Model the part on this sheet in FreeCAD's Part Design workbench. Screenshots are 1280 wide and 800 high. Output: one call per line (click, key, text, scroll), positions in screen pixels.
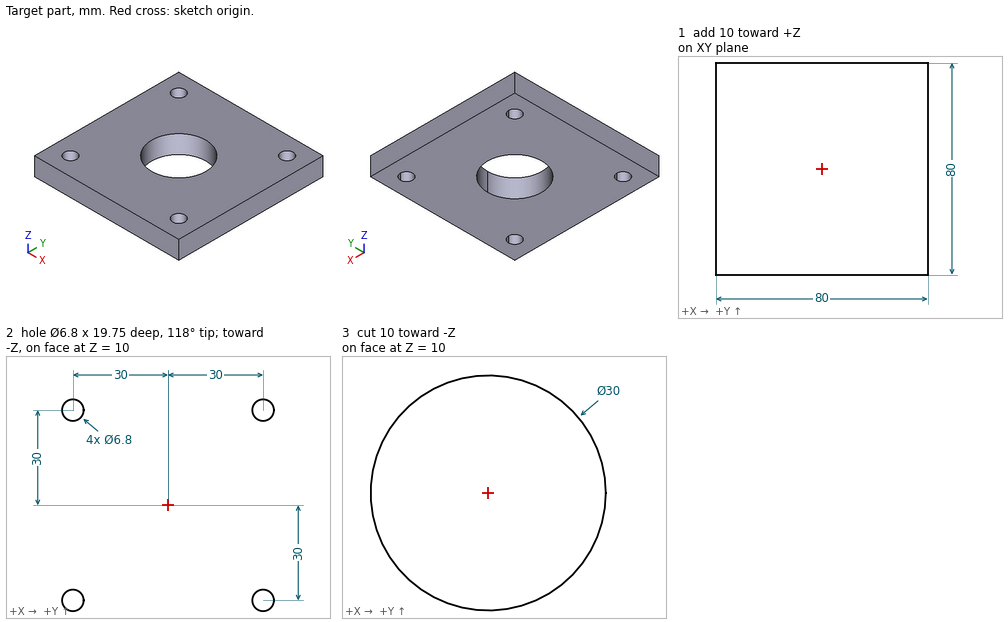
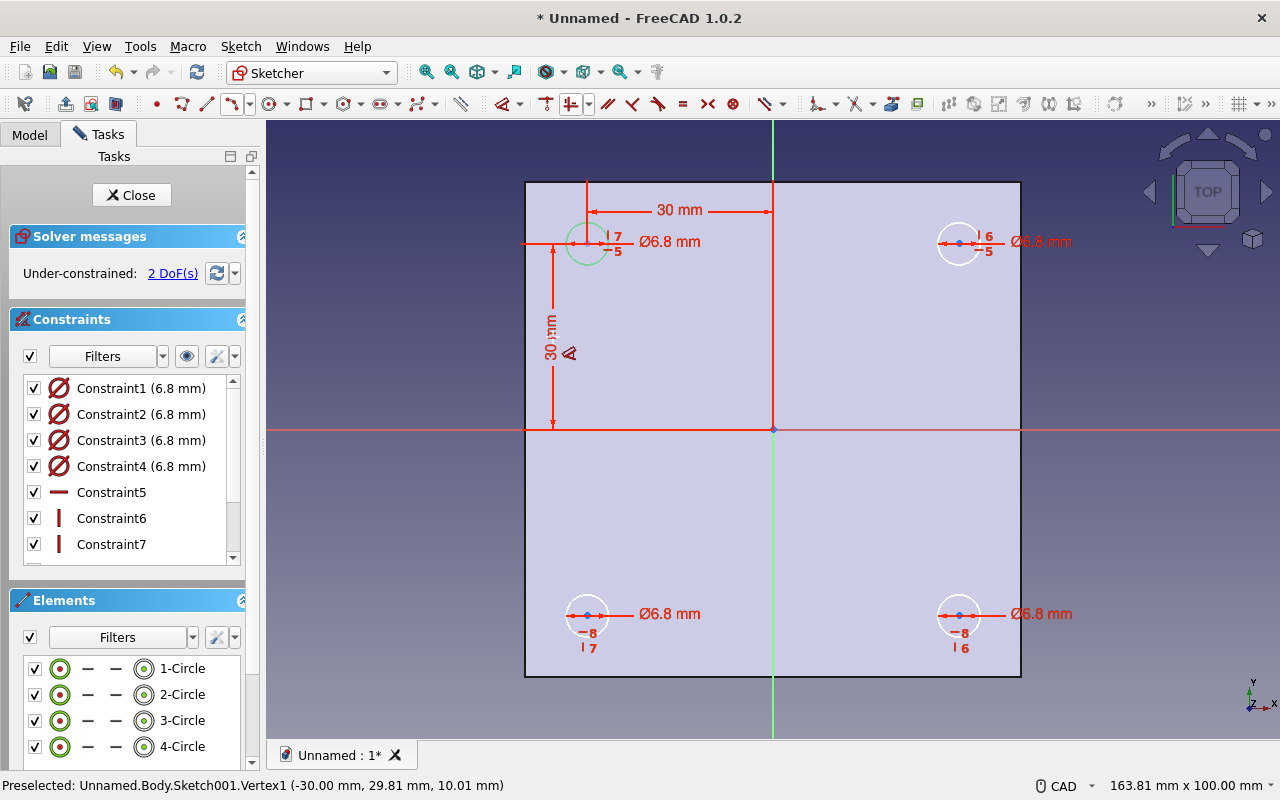
click(959, 244)
click(866, 210)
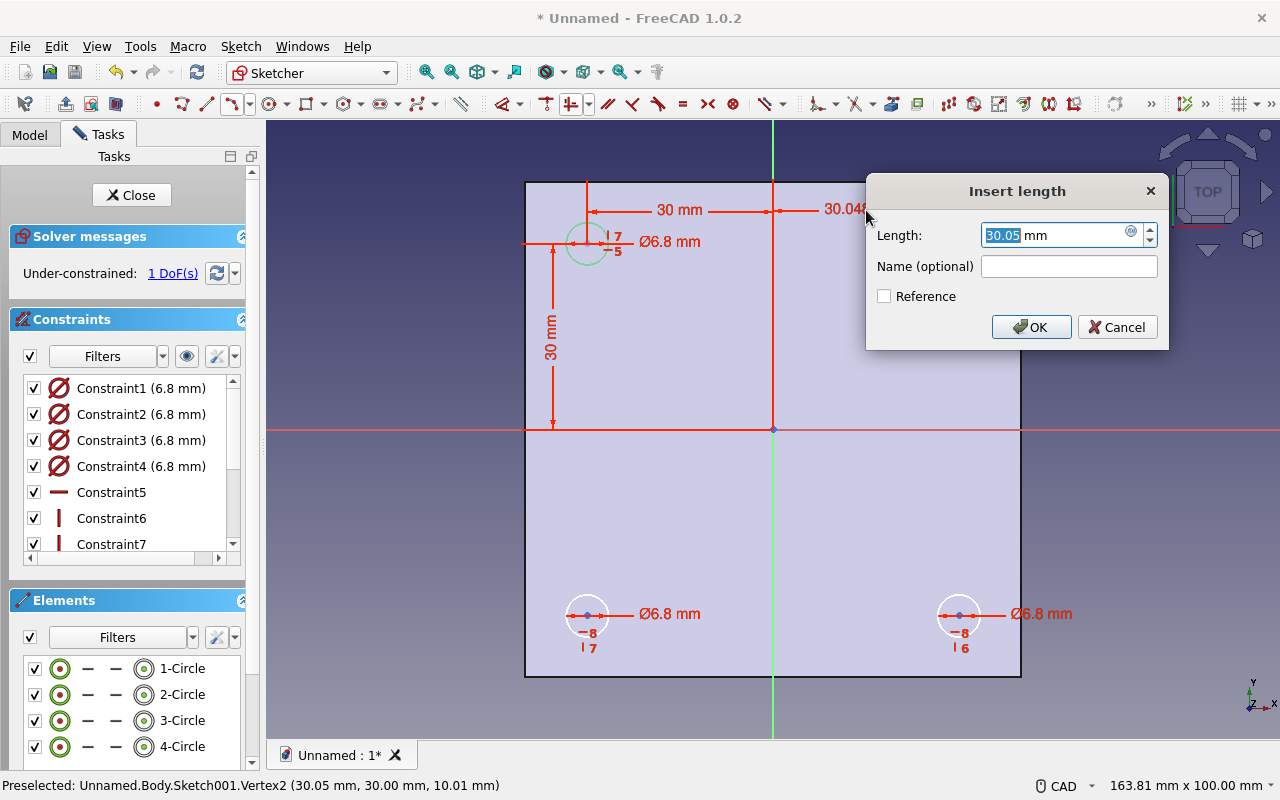
text(30)
key(Return)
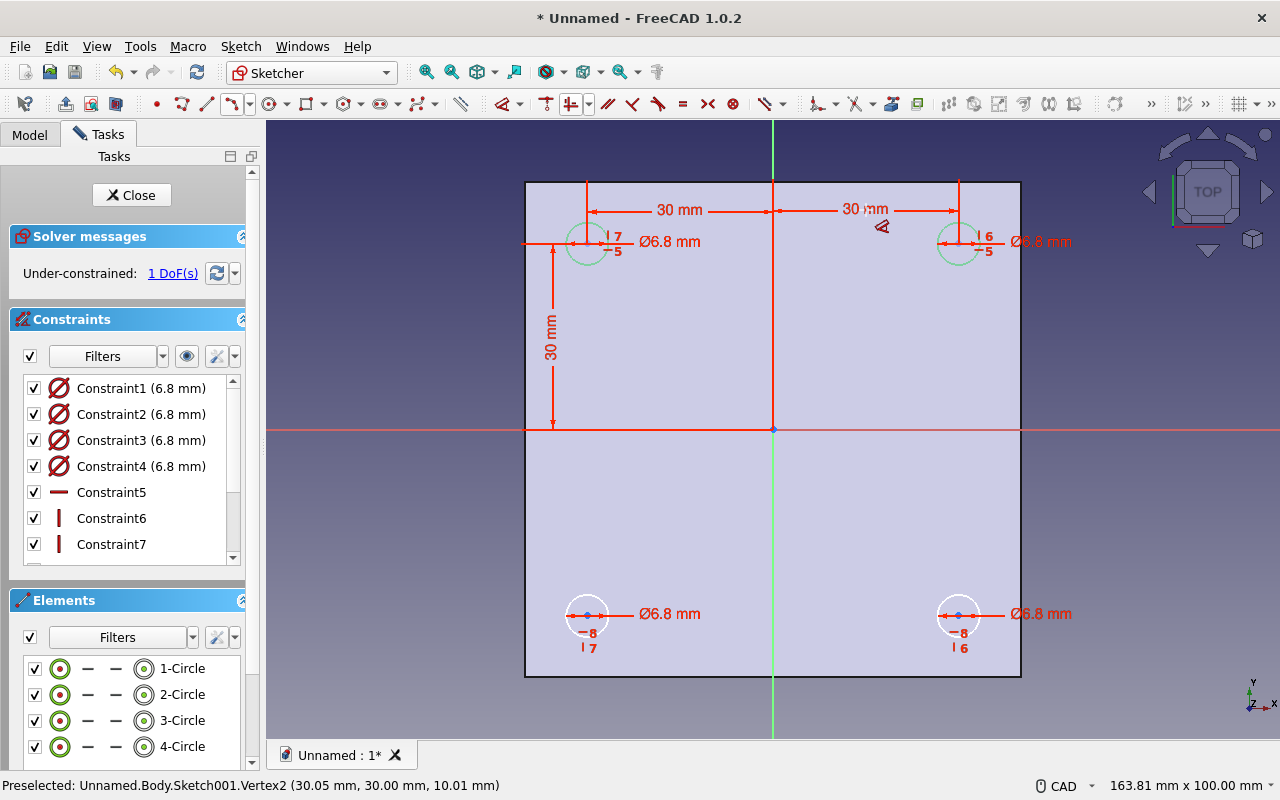
click(959, 616)
click(993, 523)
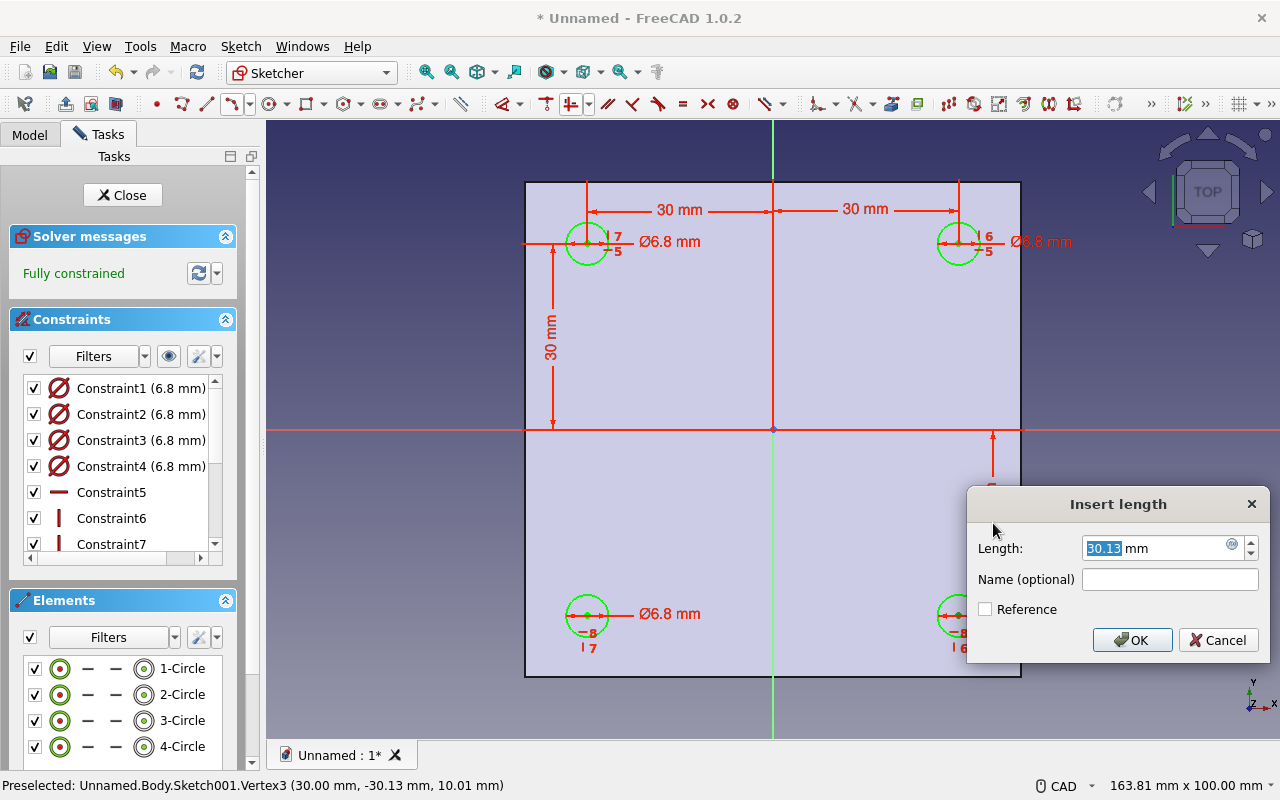
text(30)
key(Return)
key(Escape)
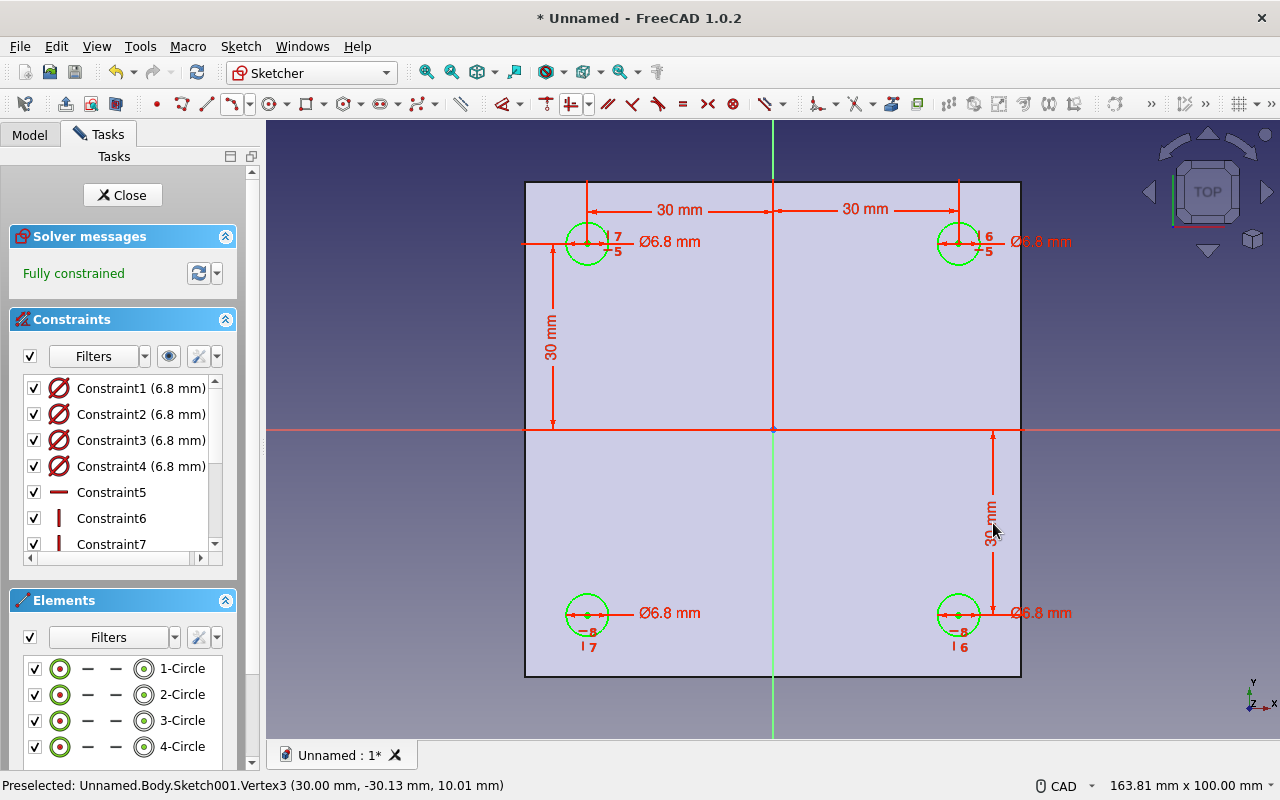
click(123, 195)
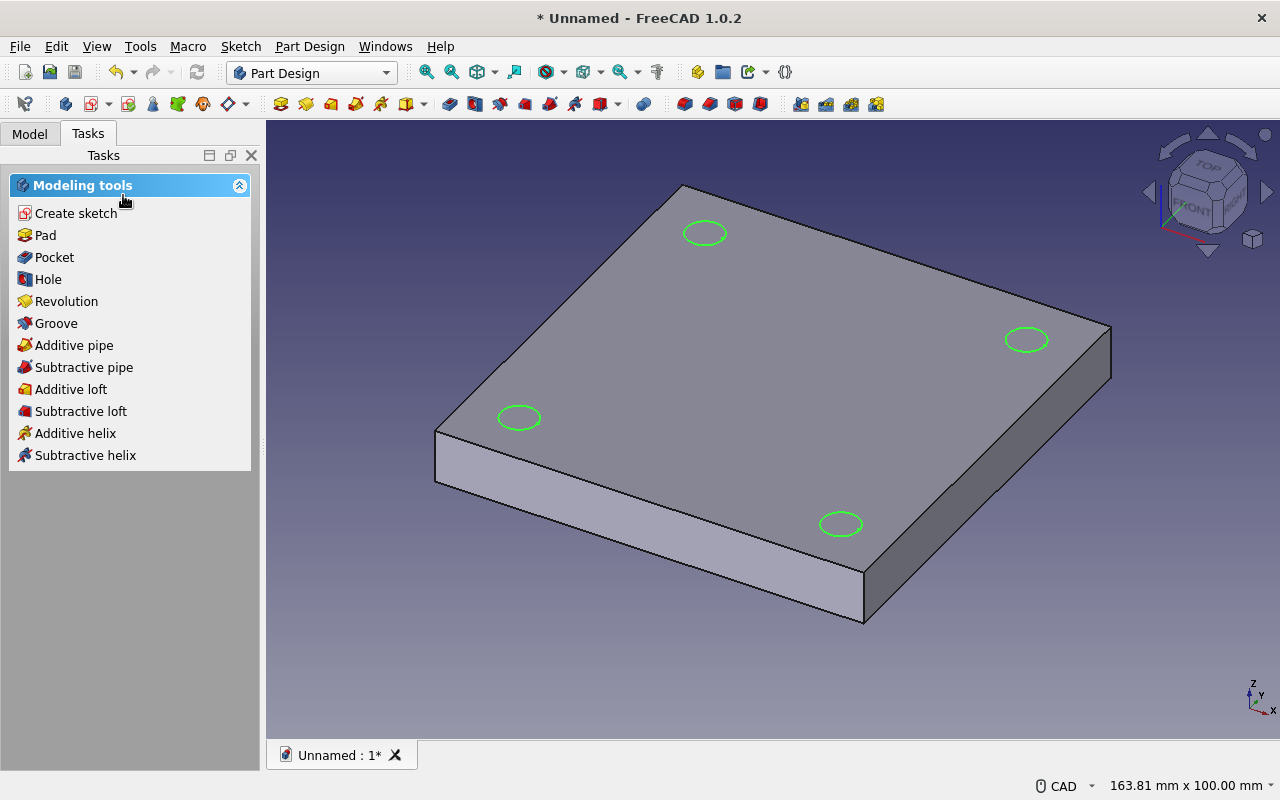
click(475, 104)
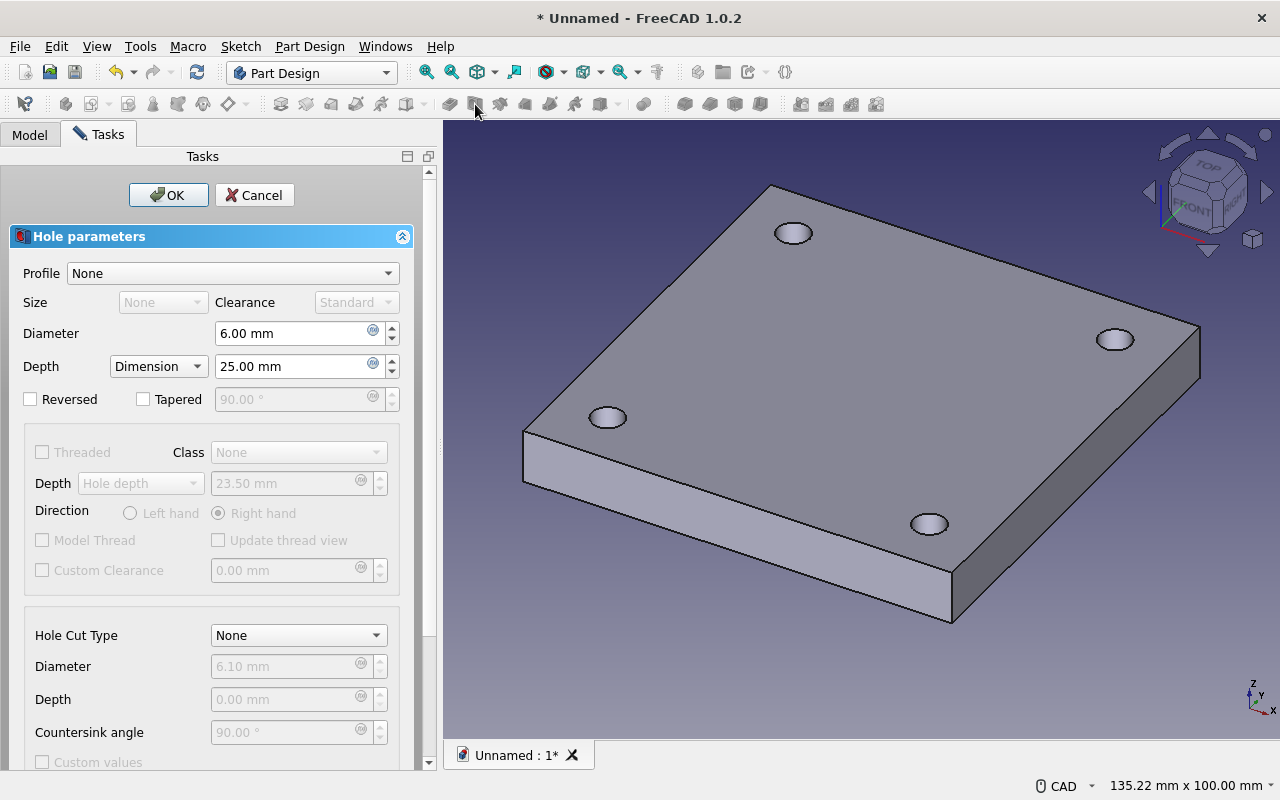
triple_click(300, 334)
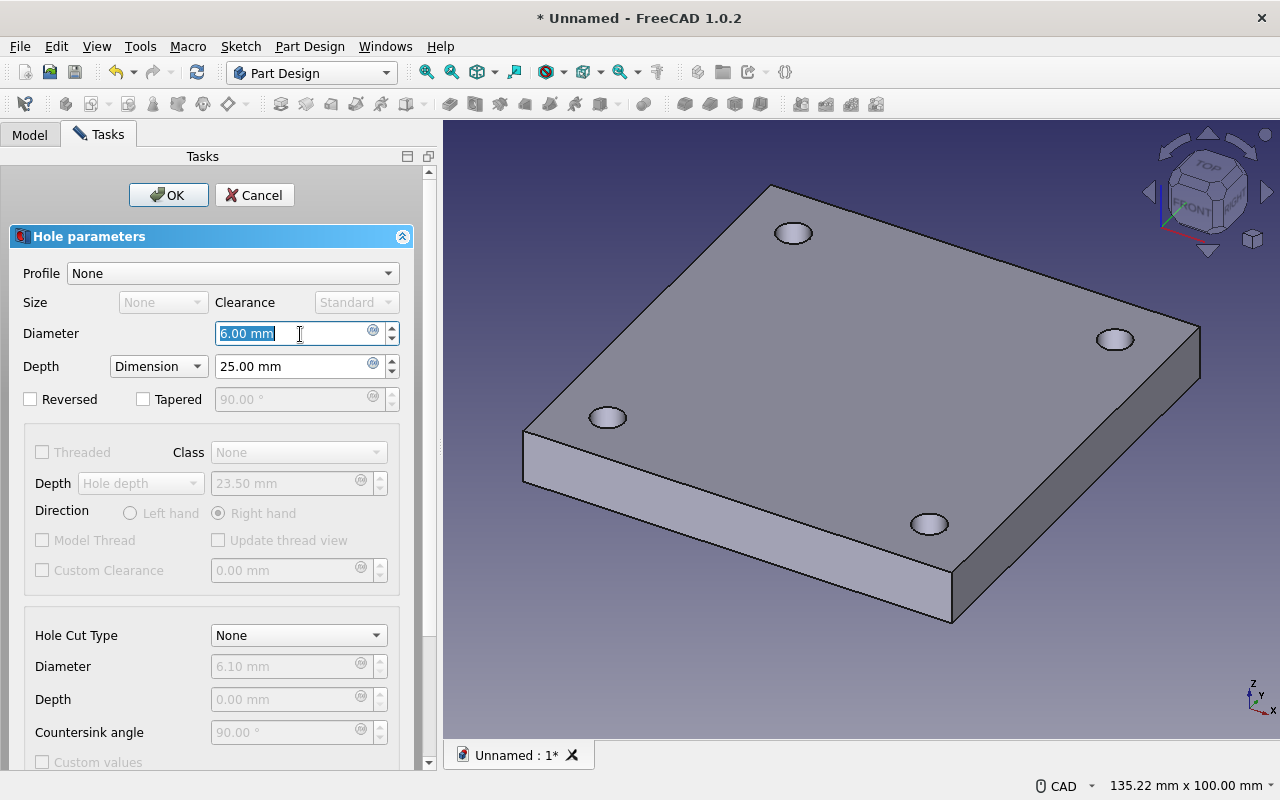
text(6.8)
key(Tab)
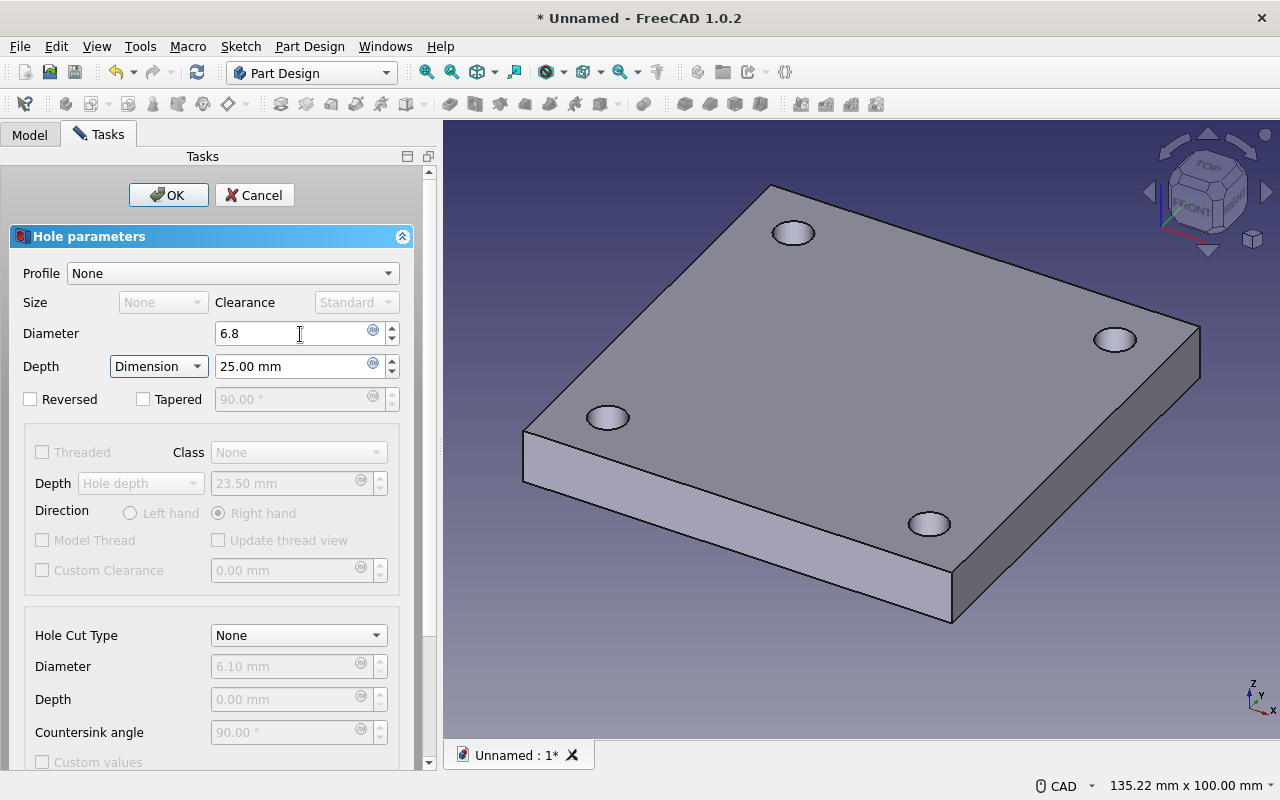
triple_click(300, 366)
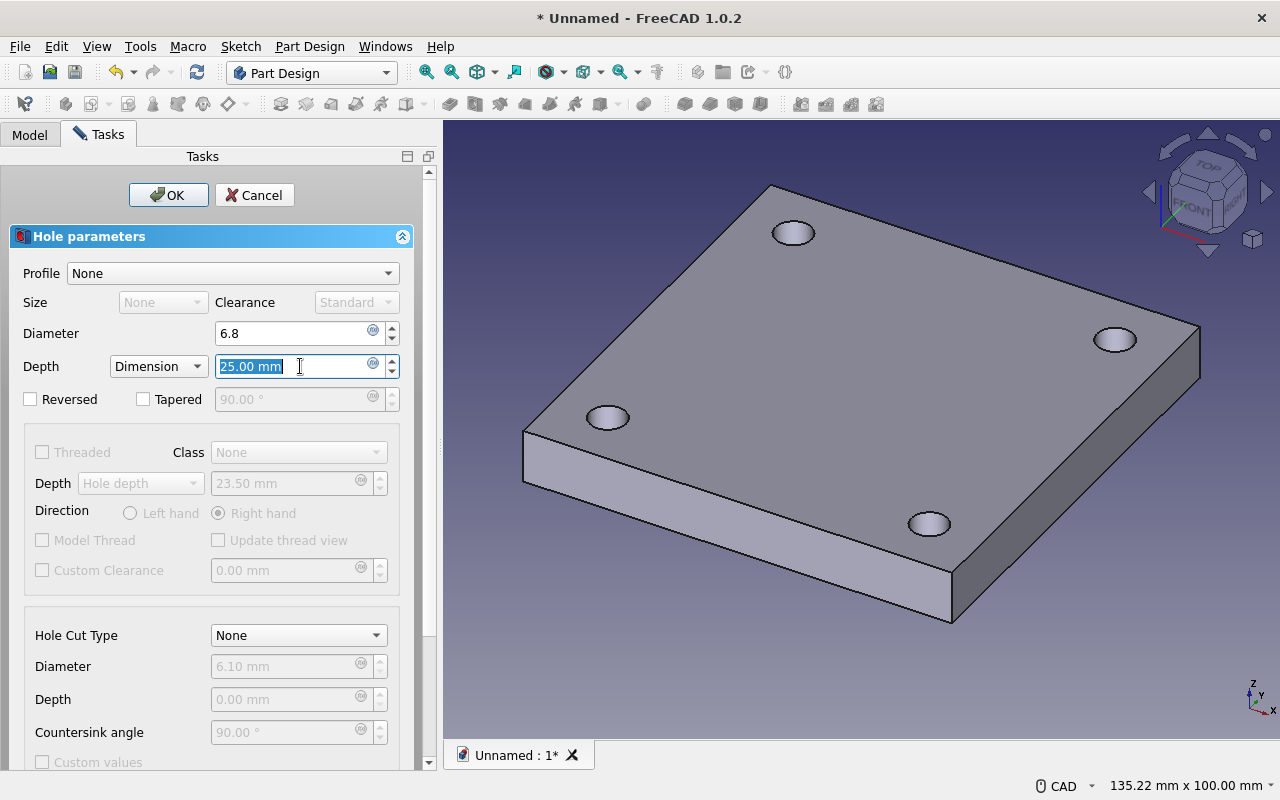
text(19.75)
key(Tab)